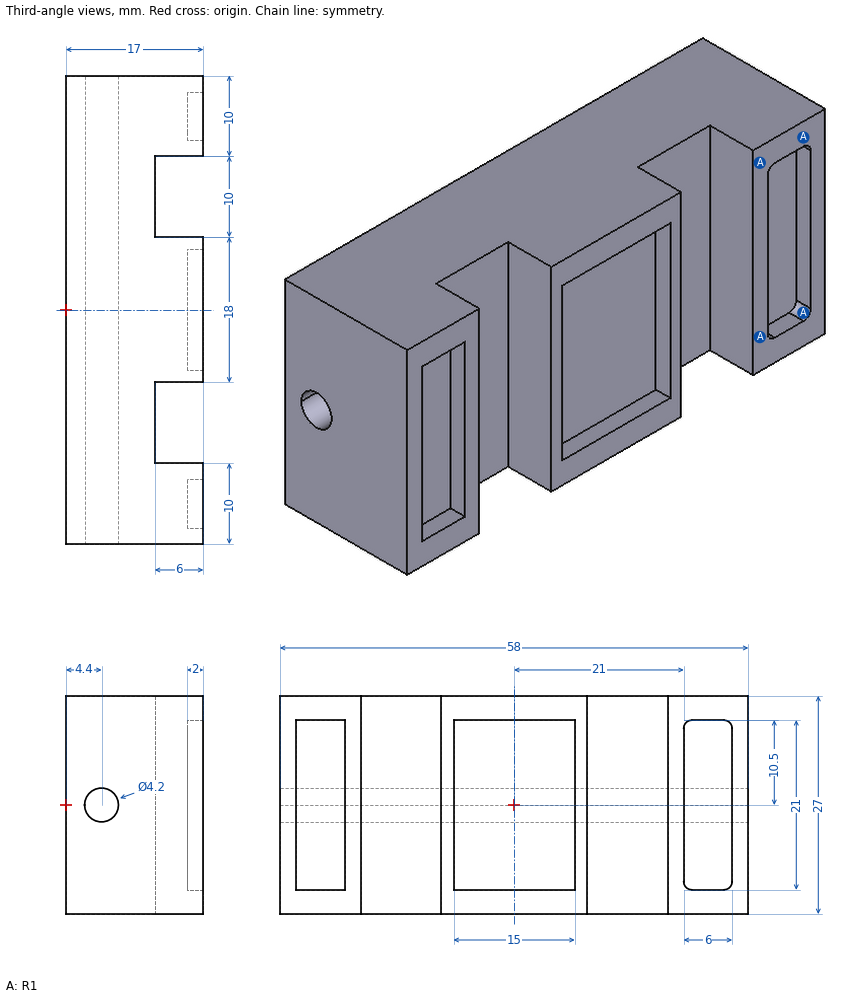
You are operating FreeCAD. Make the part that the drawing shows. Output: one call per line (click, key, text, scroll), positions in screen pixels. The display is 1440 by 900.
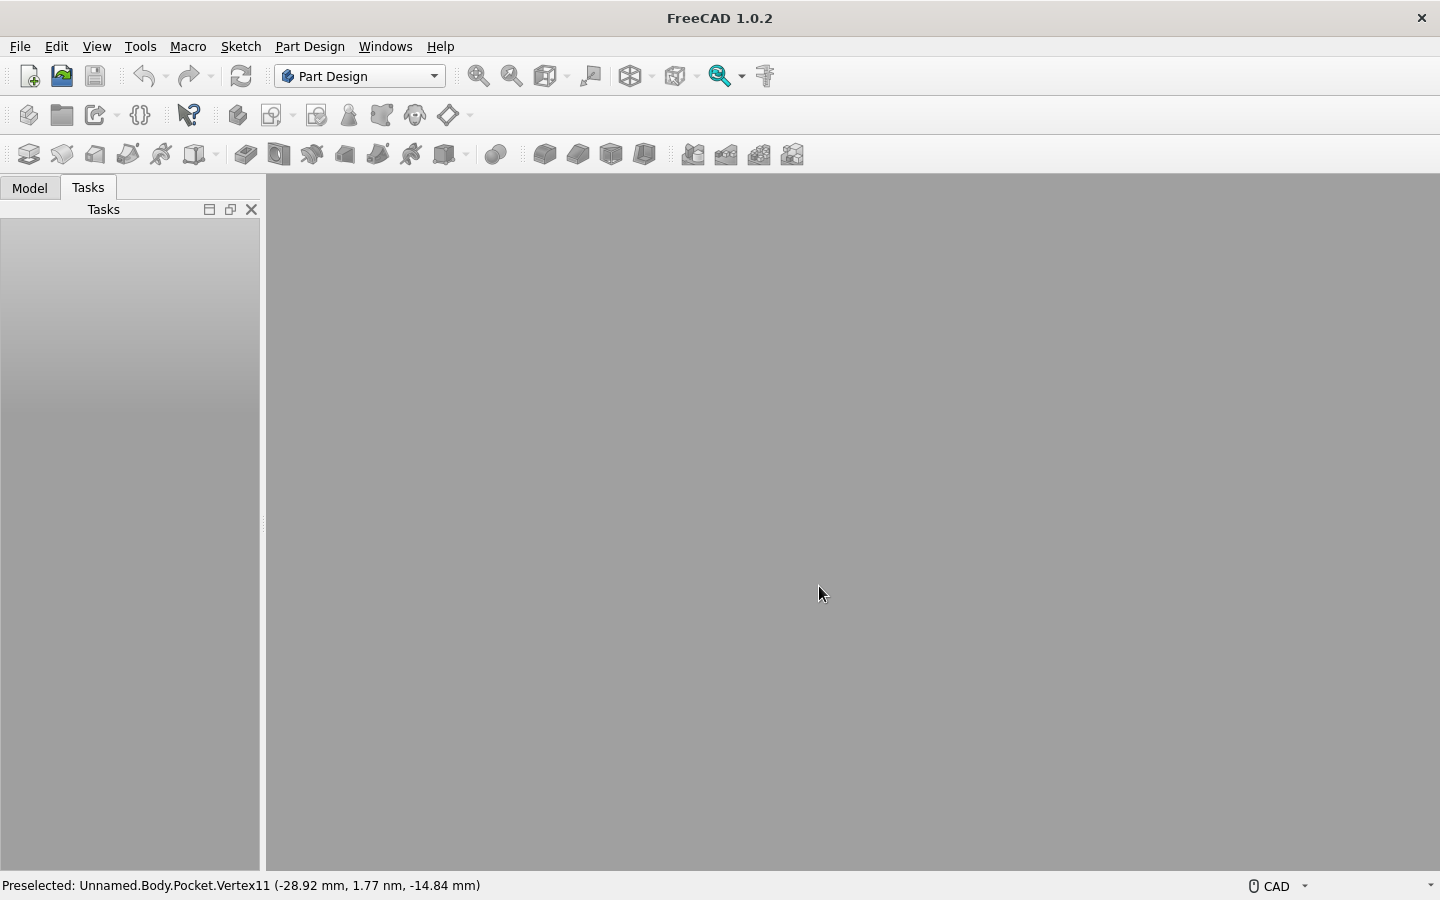
click(29, 76)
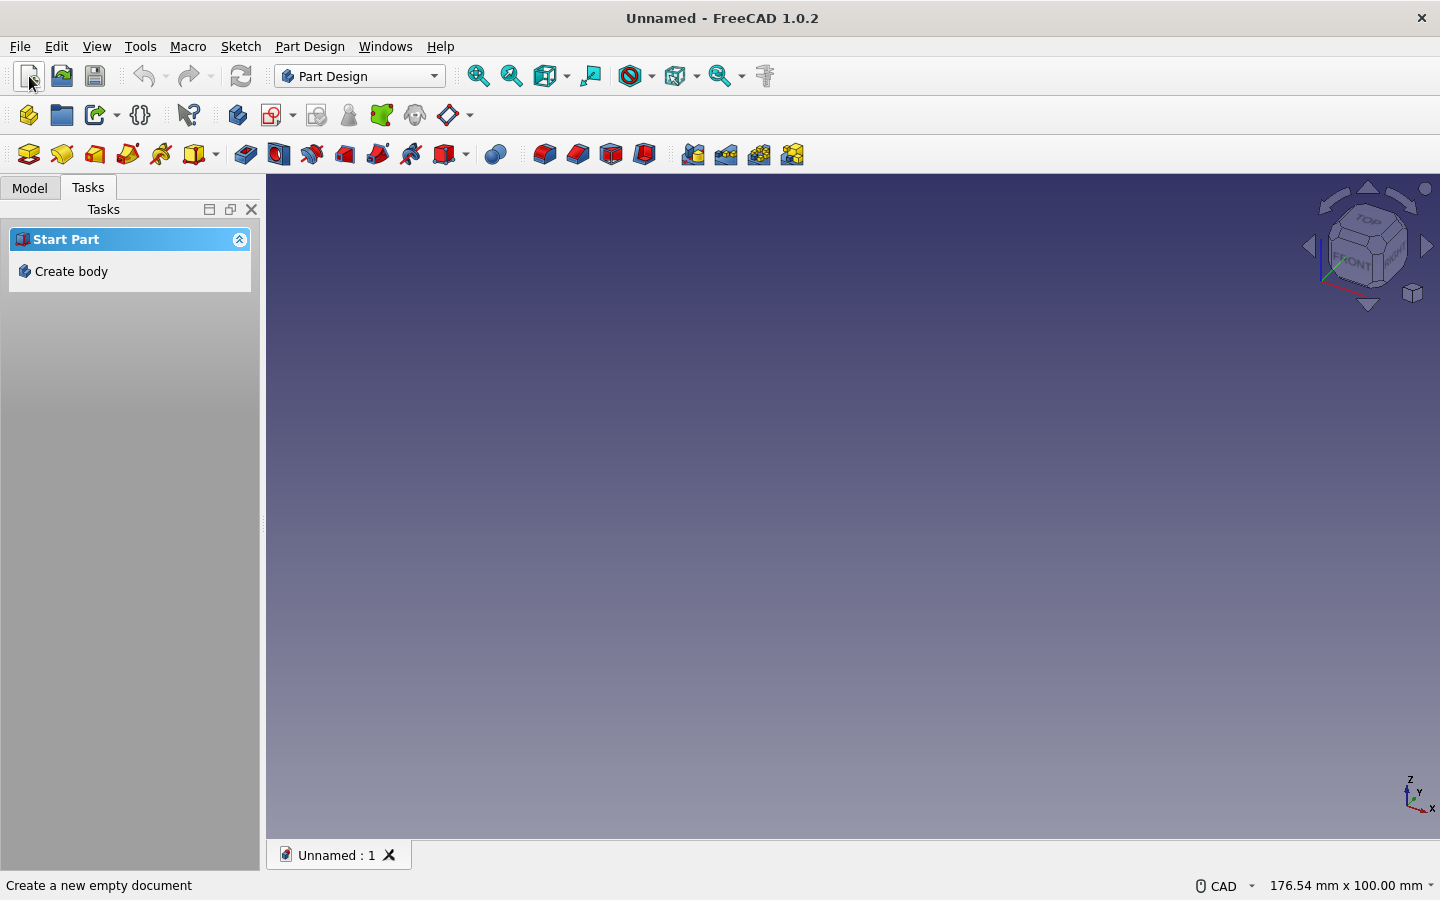
click(270, 116)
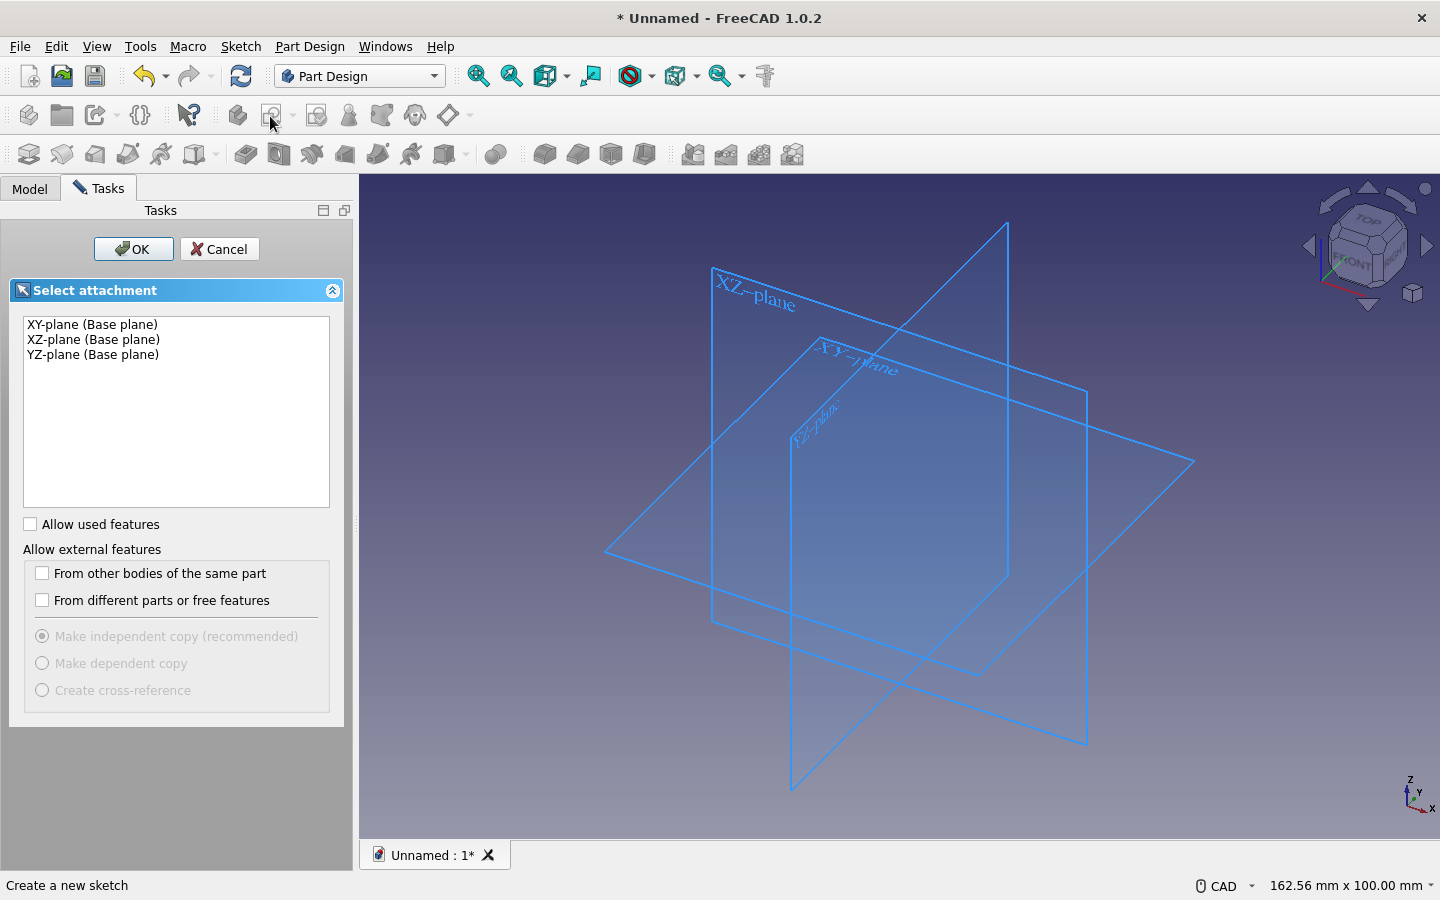
click(84, 324)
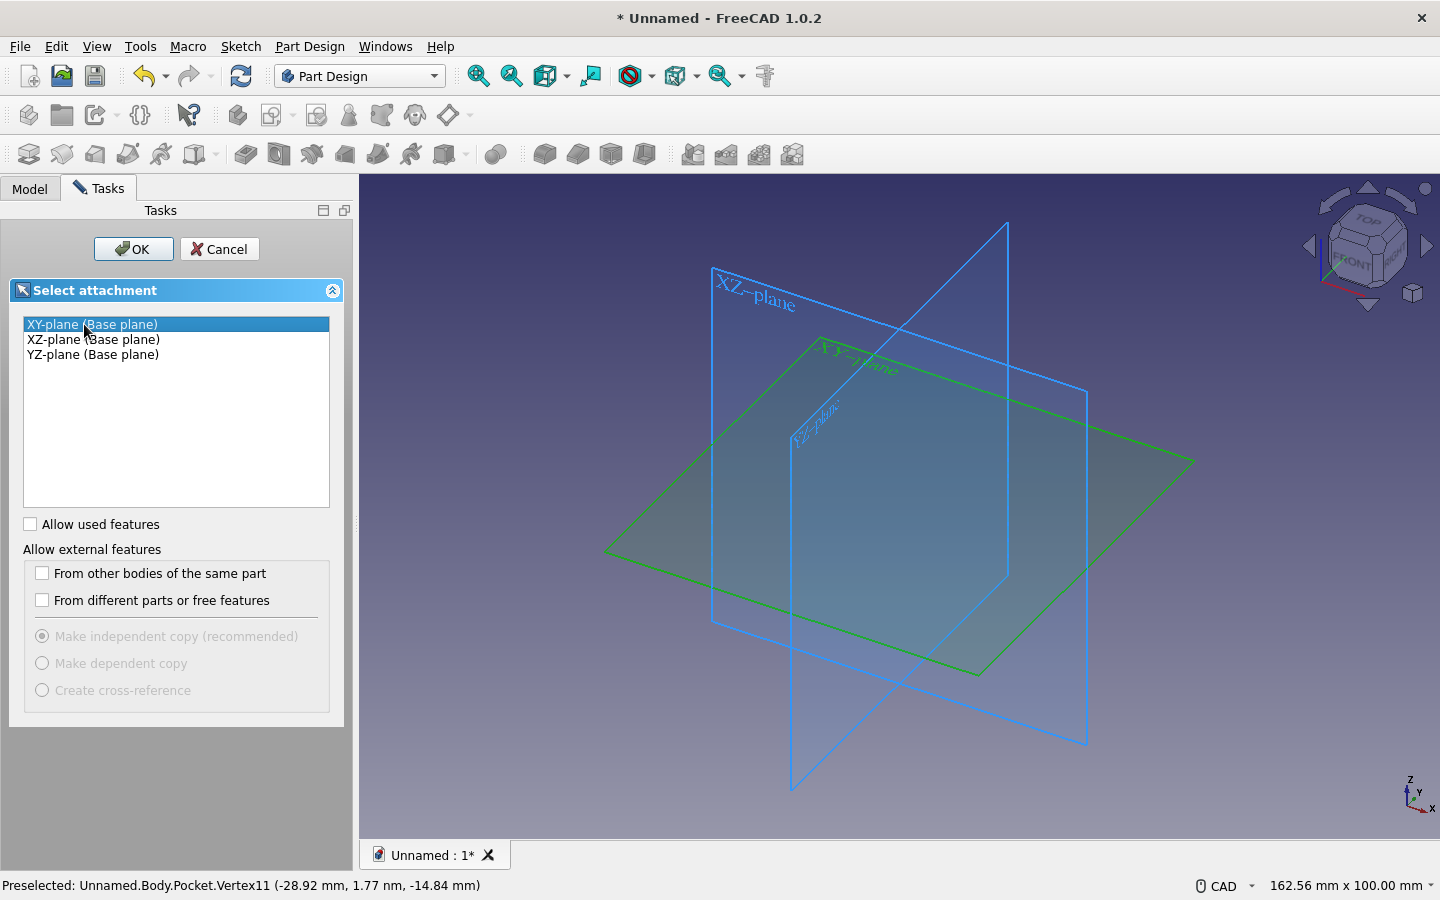
click(134, 249)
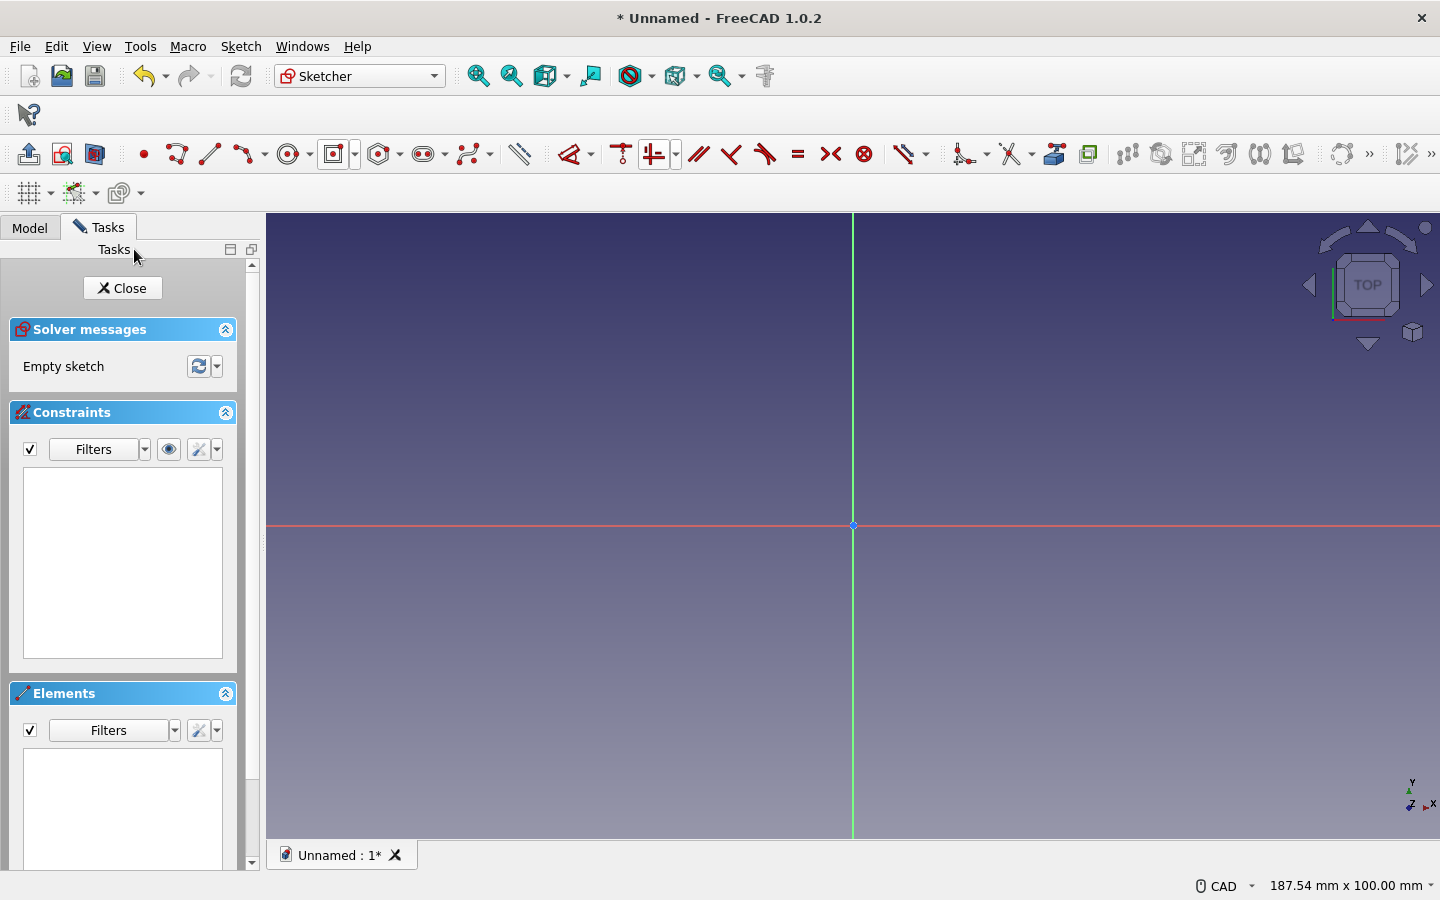
click(177, 154)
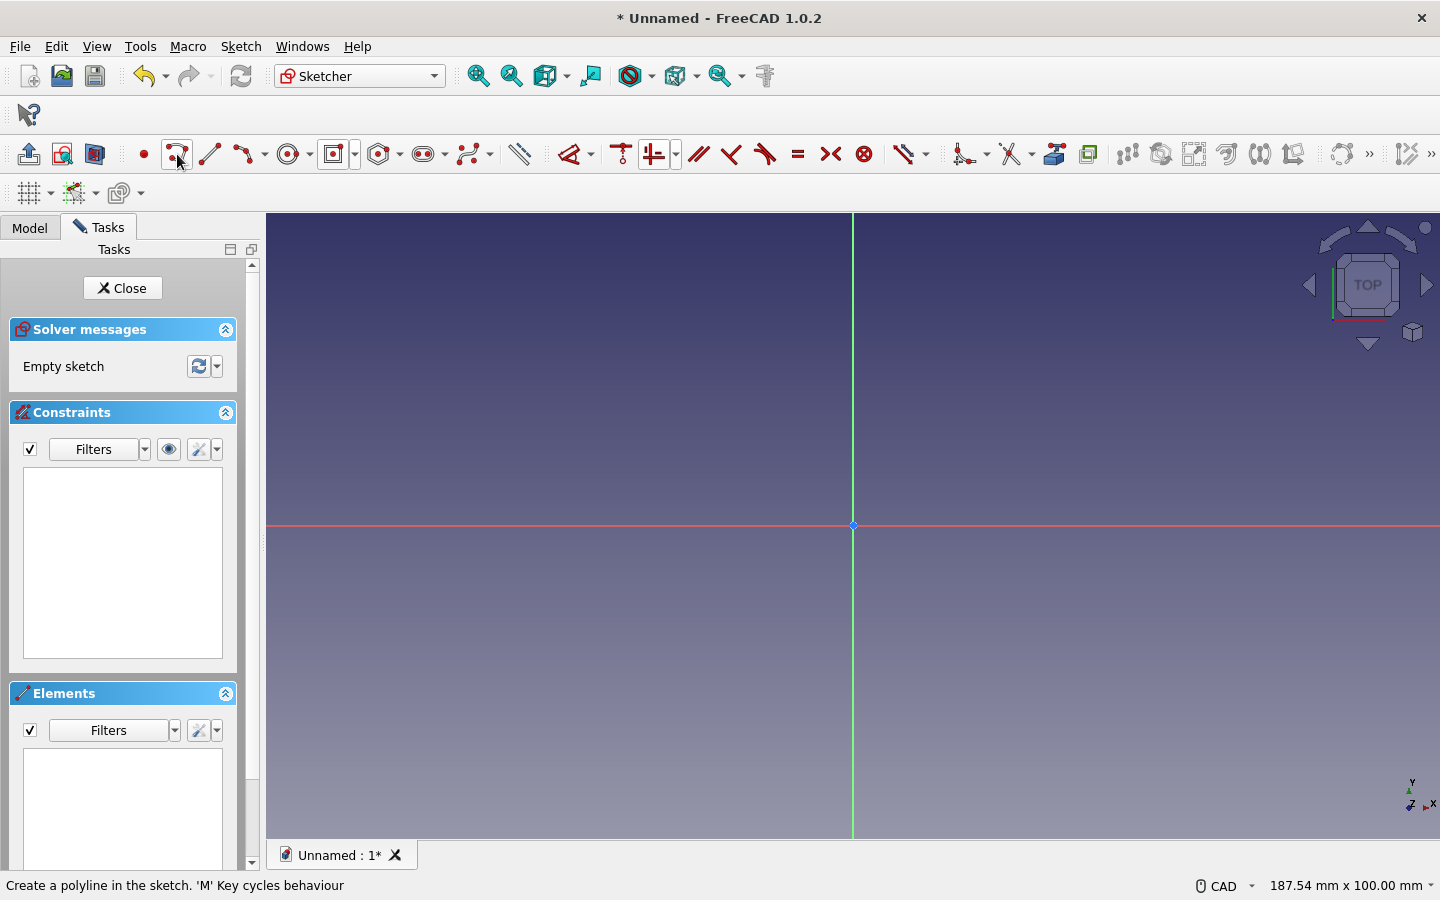
click(922, 582)
click(959, 582)
click(959, 470)
click(922, 470)
click(922, 407)
click(959, 407)
click(959, 344)
click(853, 344)
click(862, 708)
click(959, 708)
click(959, 645)
click(922, 645)
click(922, 583)
key(Escape)
key(Escape)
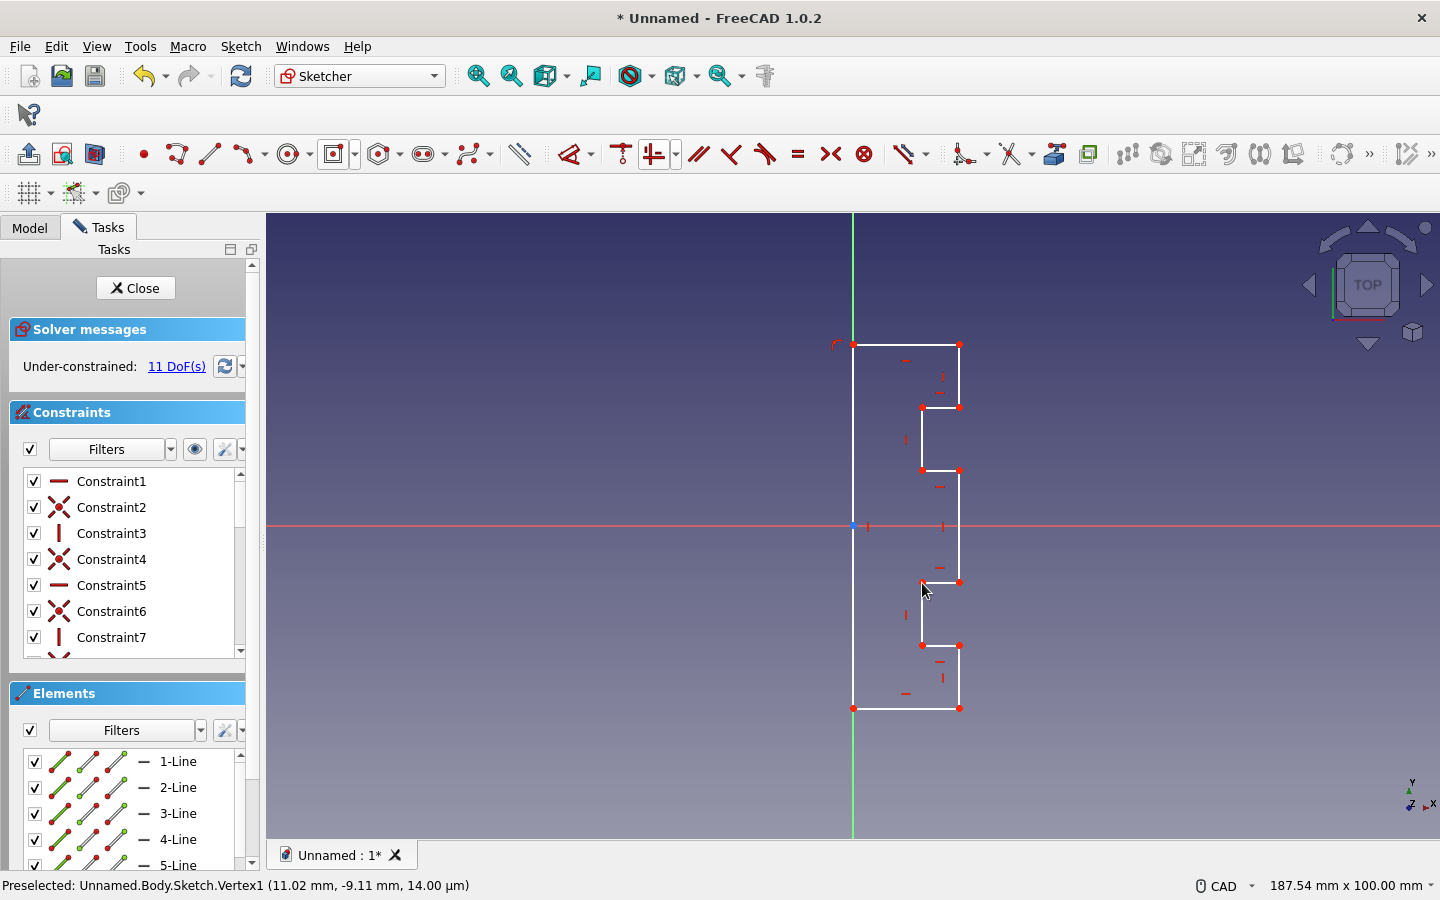
click(922, 583)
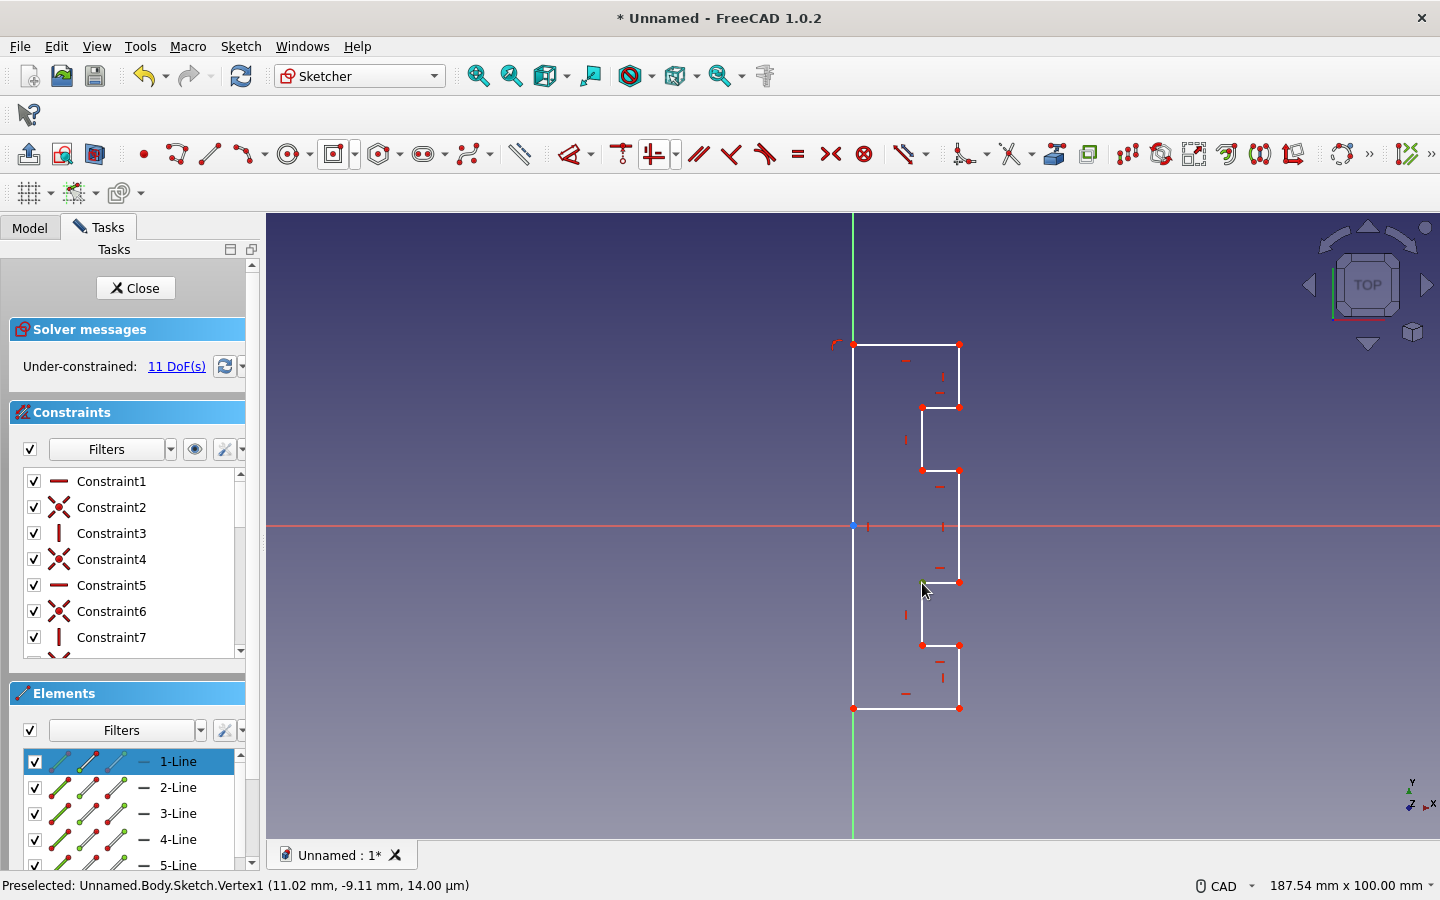
click(922, 471)